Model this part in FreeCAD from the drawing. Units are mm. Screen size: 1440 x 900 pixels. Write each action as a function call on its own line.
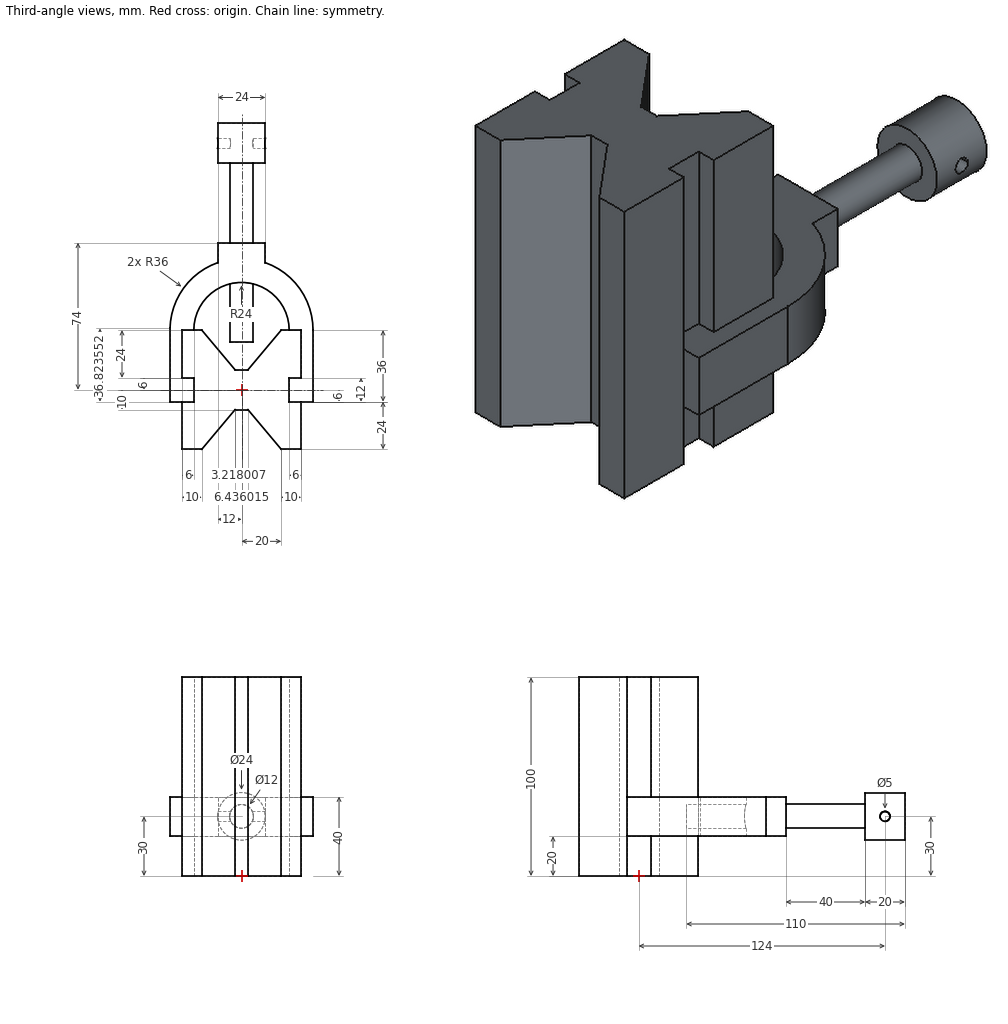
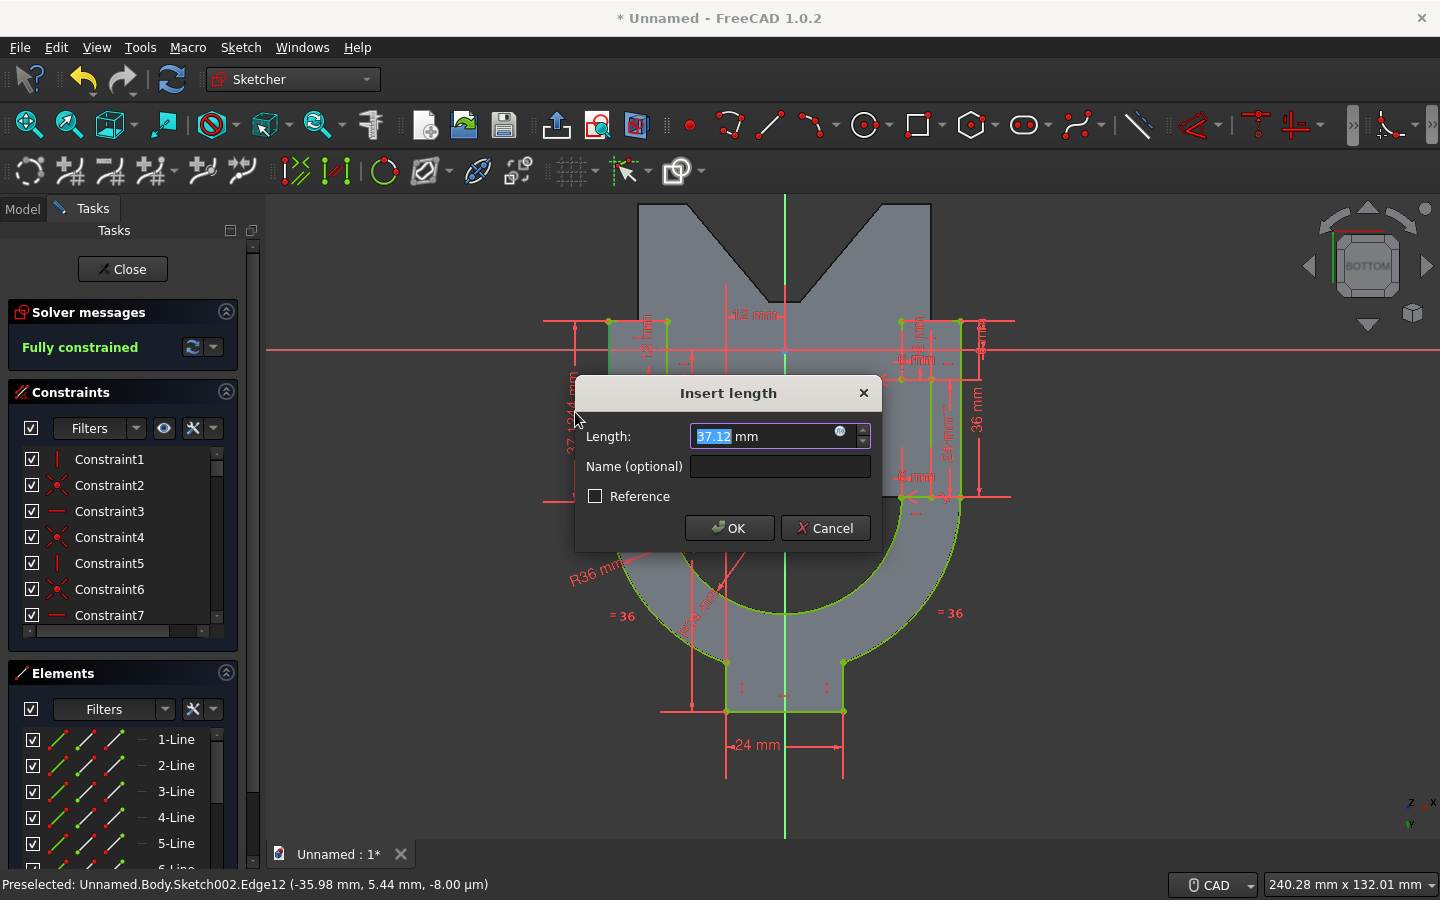
text(36.823552)
key(Return)
key(Escape)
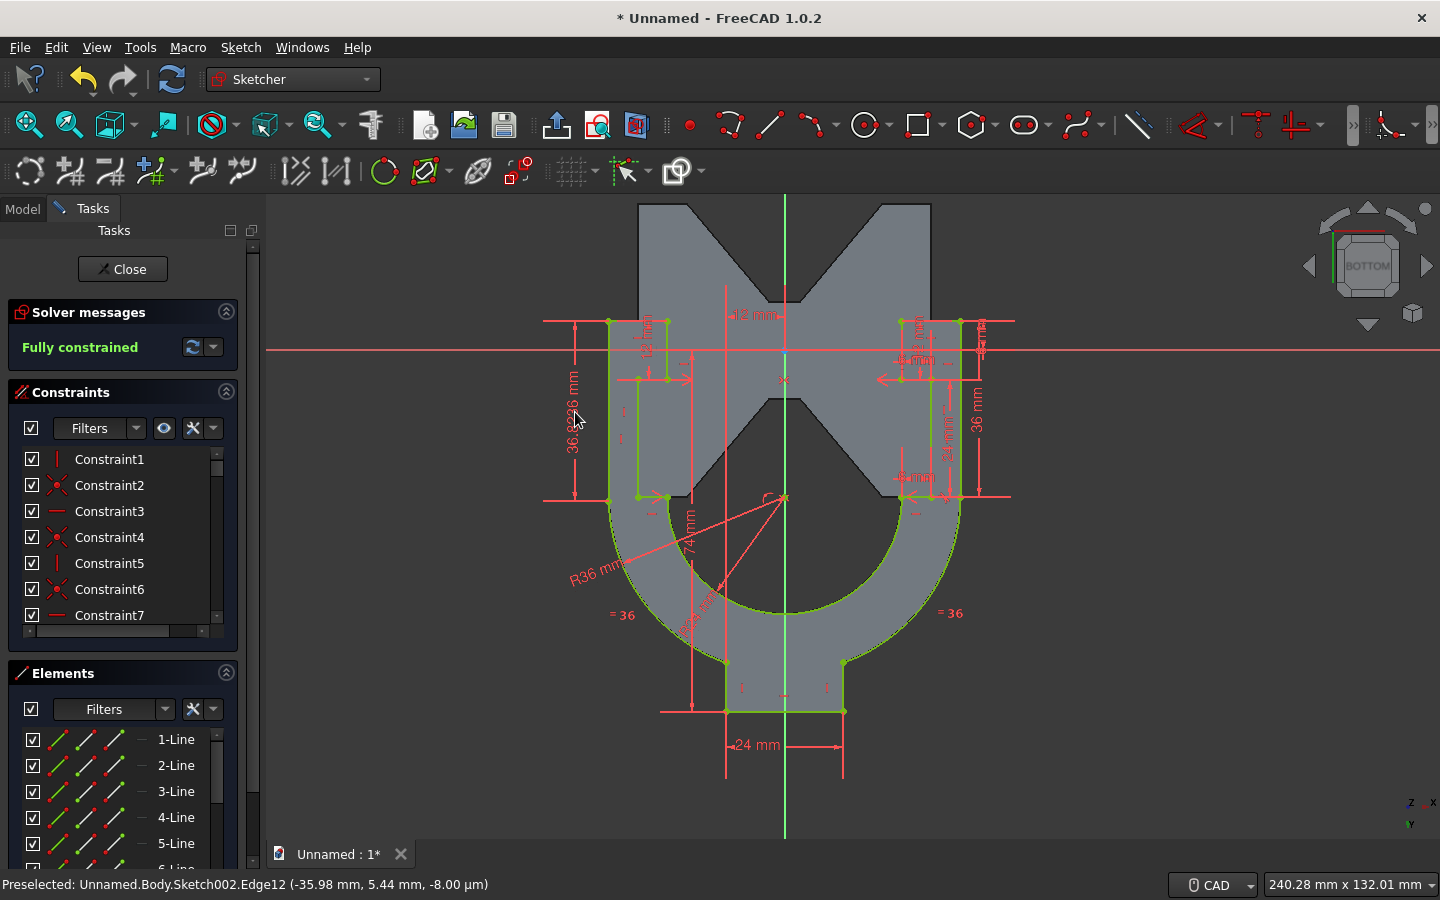
click(123, 269)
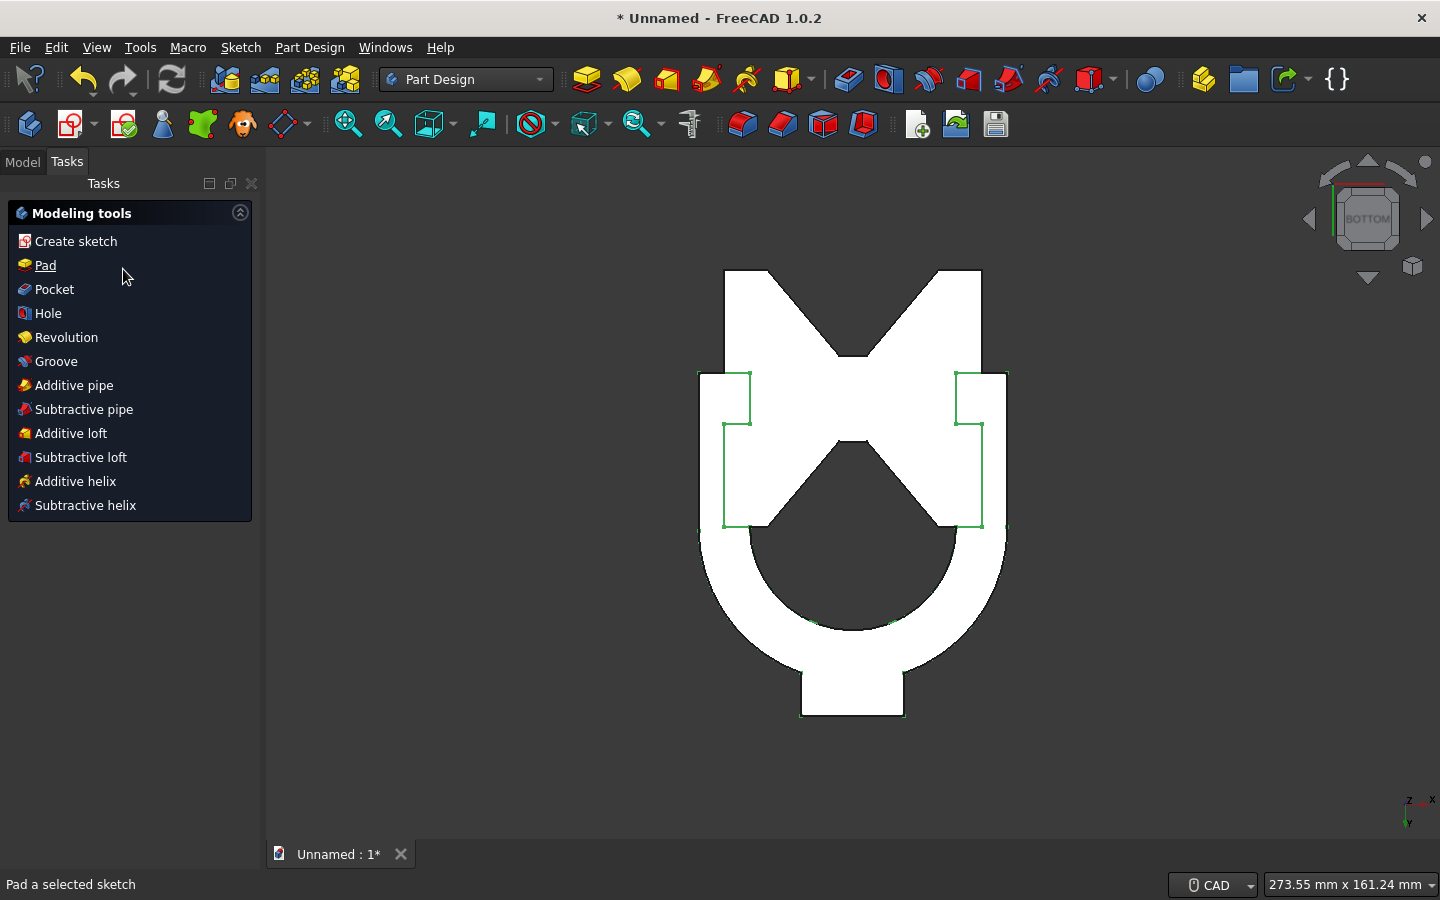
click(850, 80)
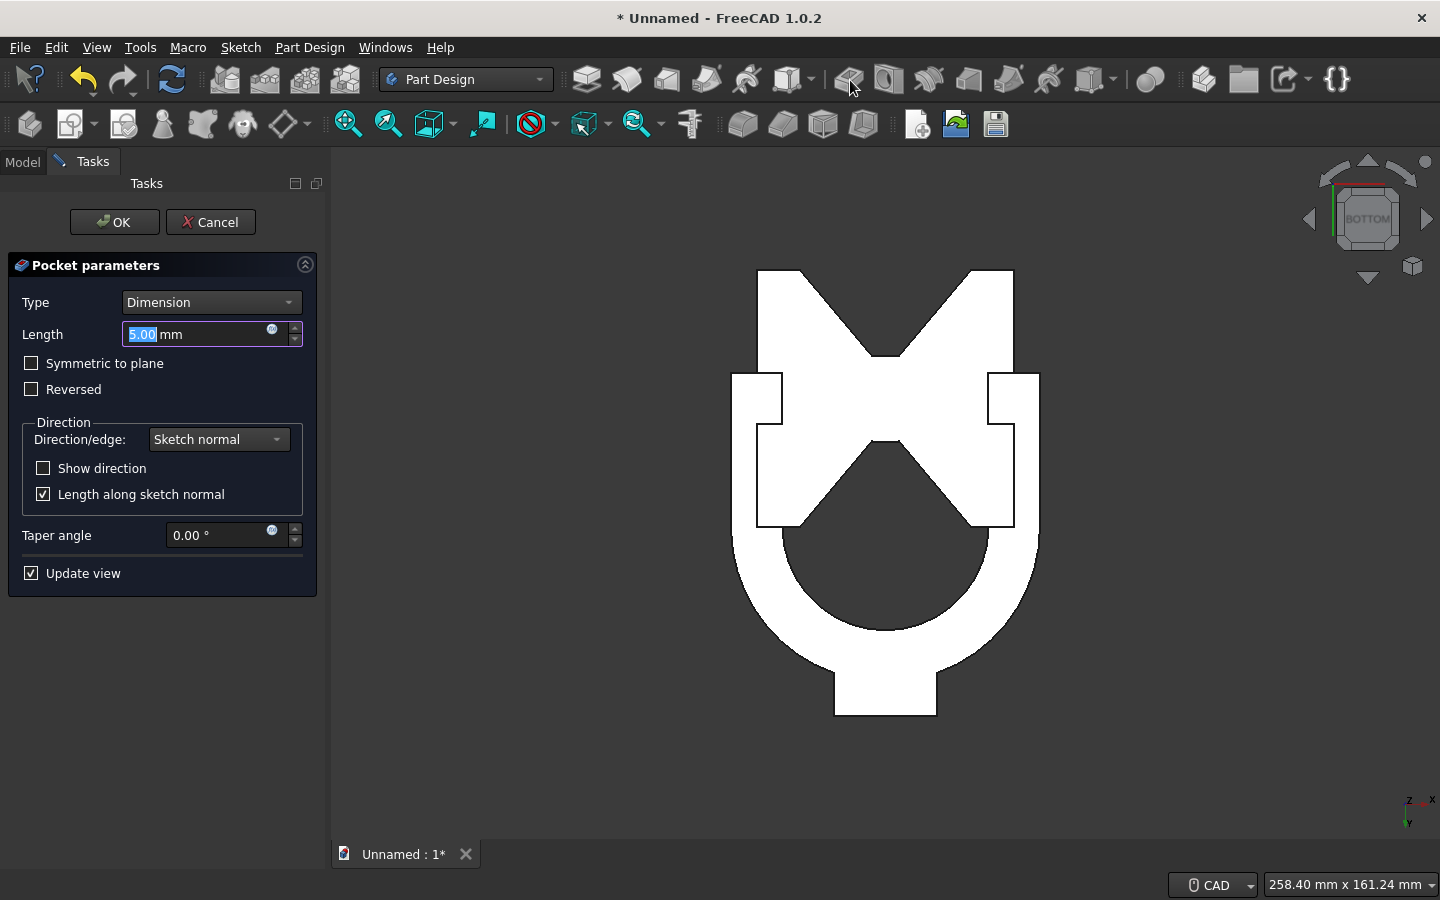
text(20)
key(Tab)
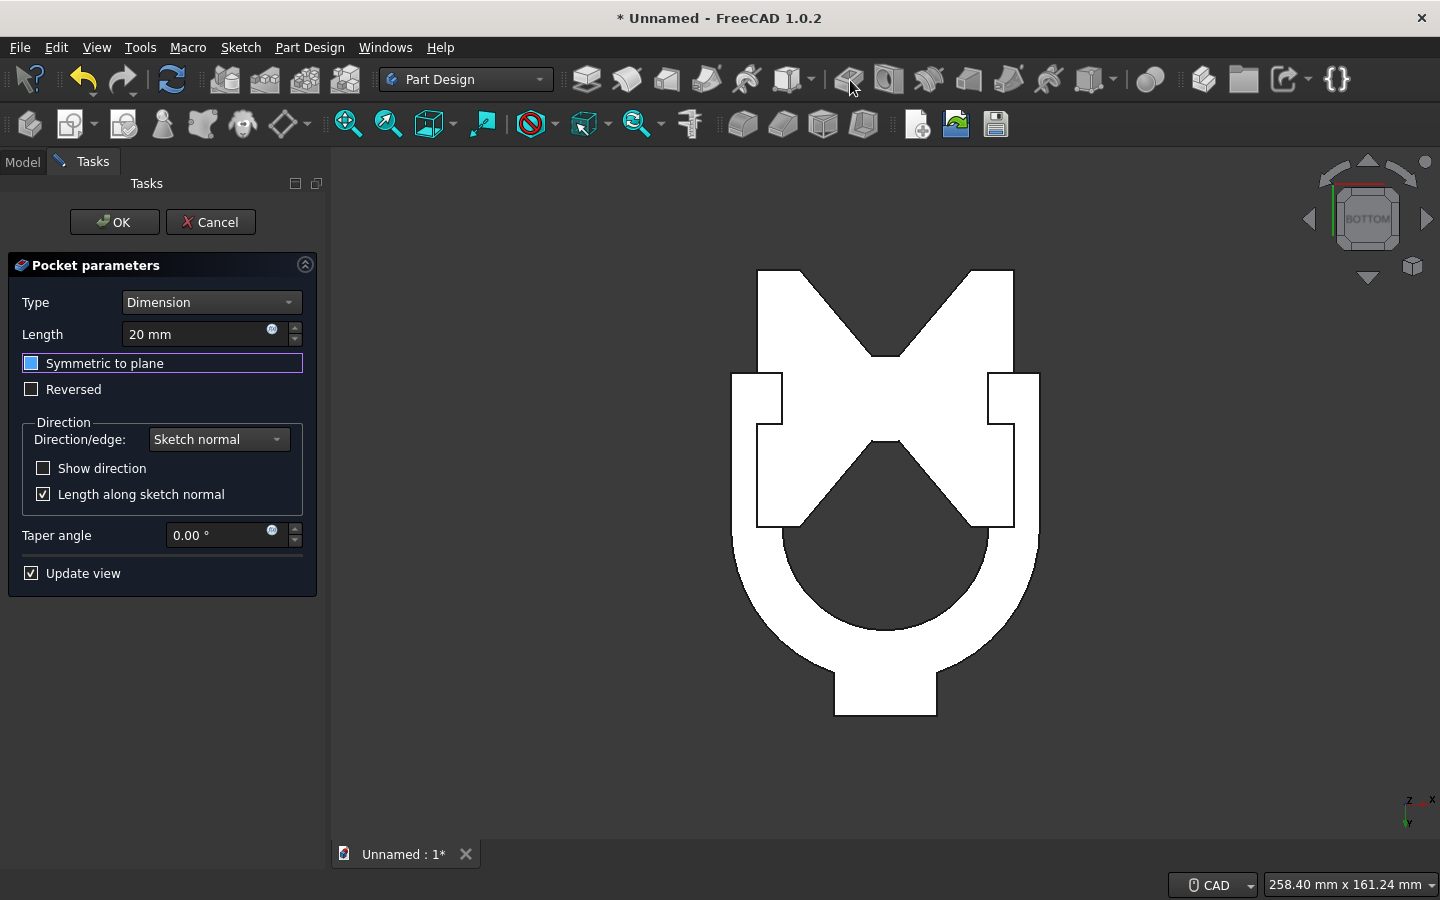
click(115, 222)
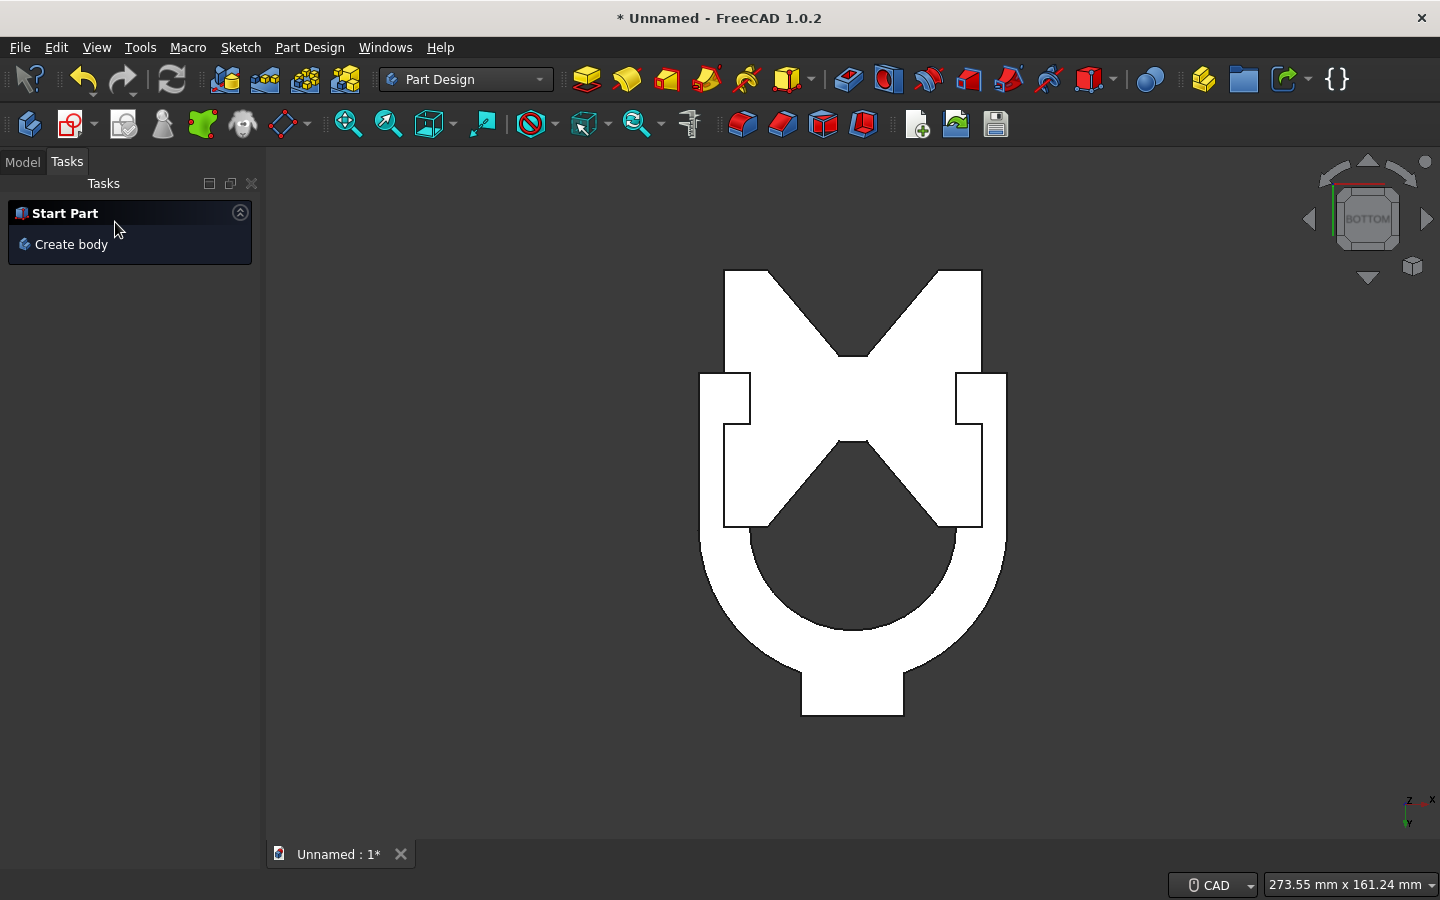
key(4)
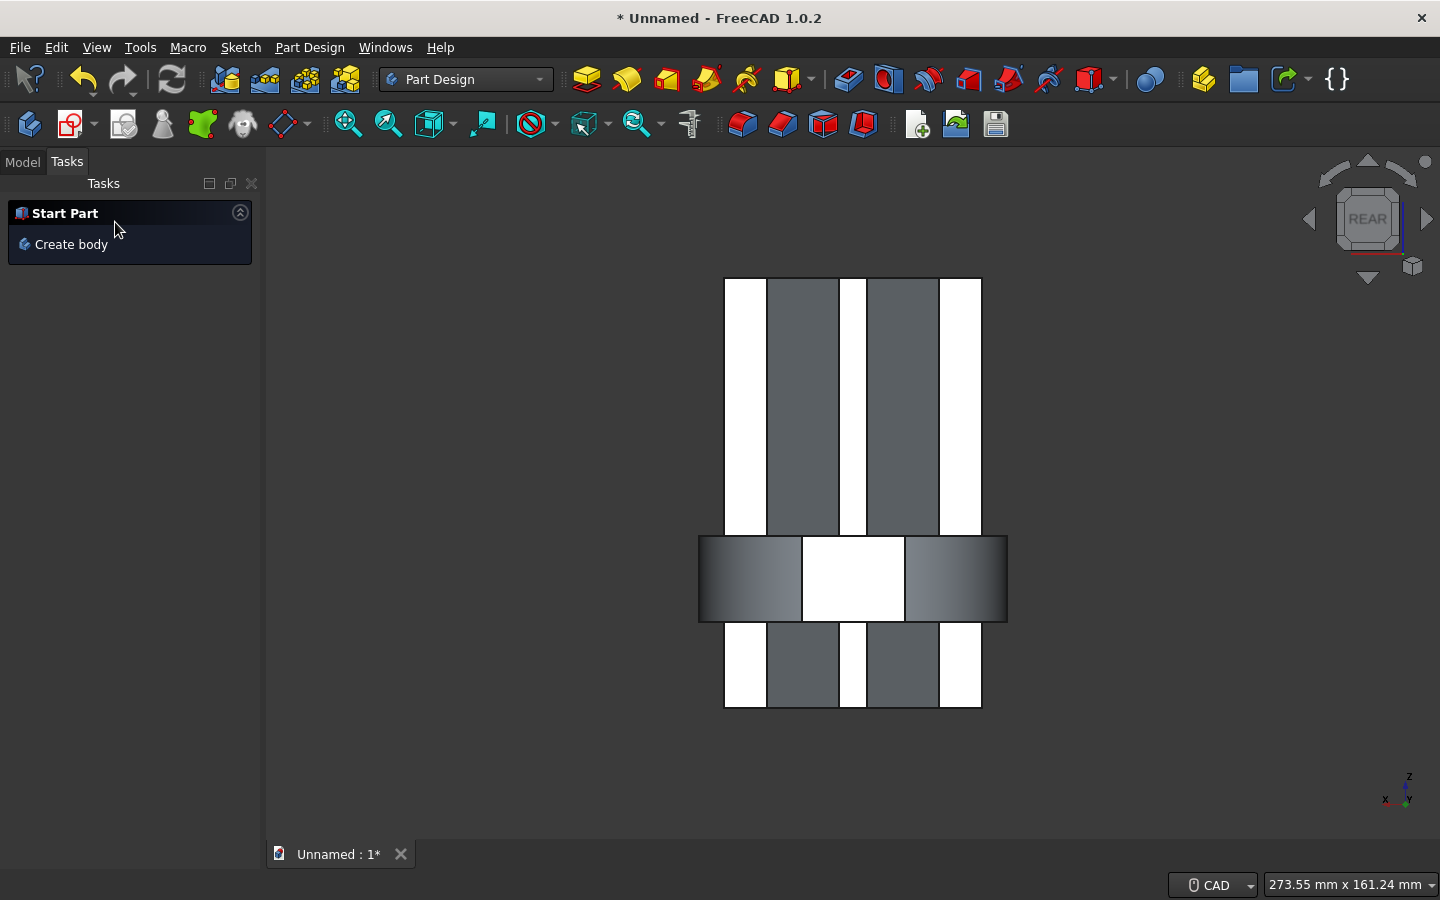
click(853, 578)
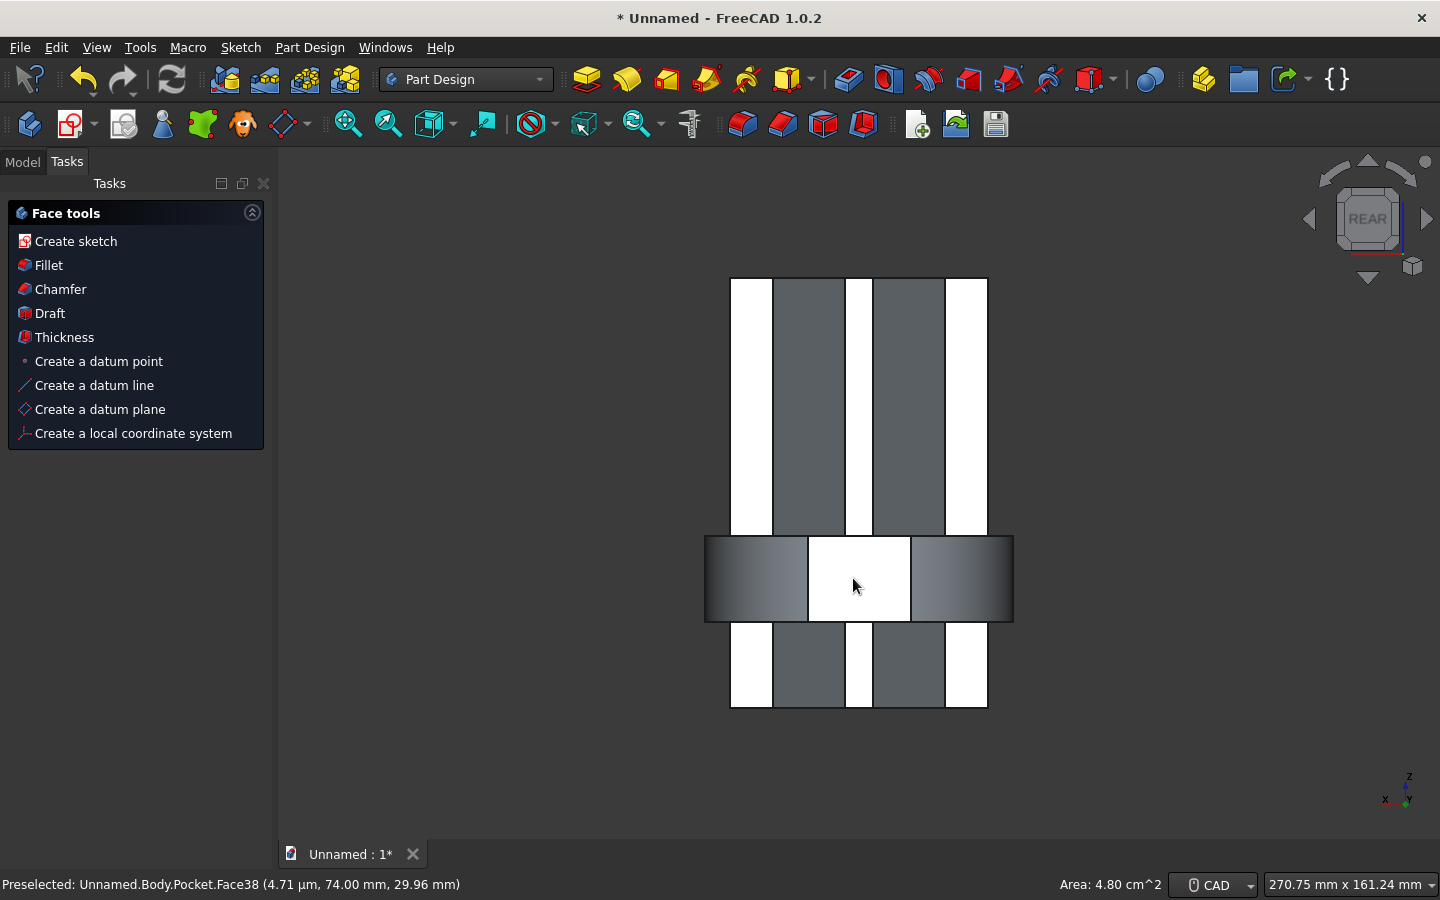
click(70, 124)